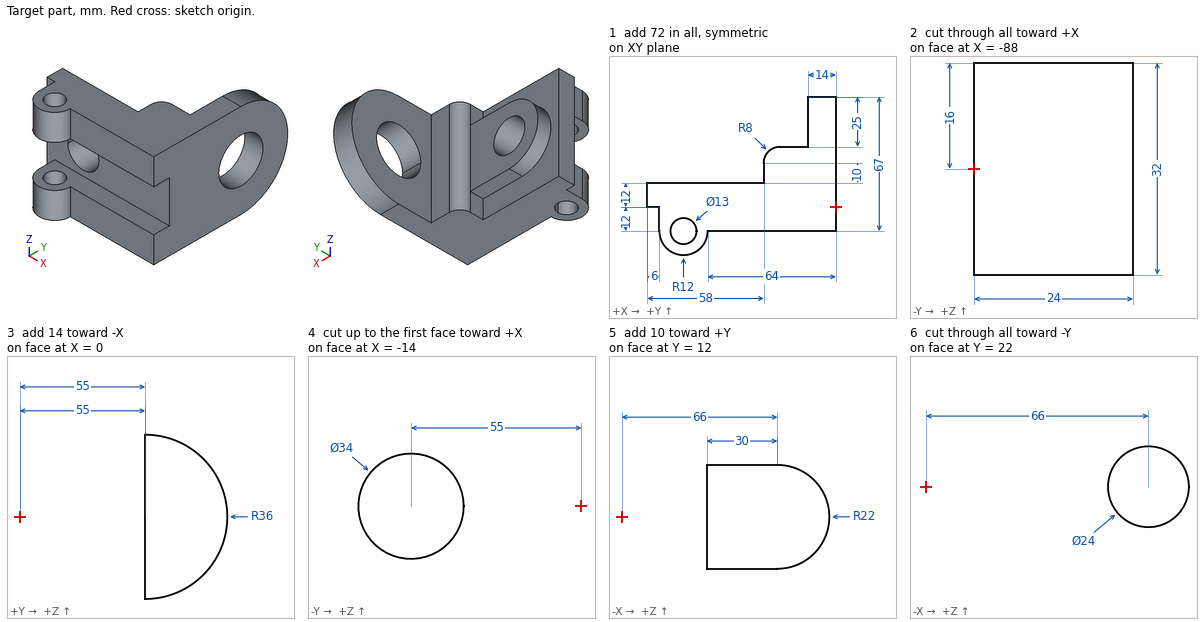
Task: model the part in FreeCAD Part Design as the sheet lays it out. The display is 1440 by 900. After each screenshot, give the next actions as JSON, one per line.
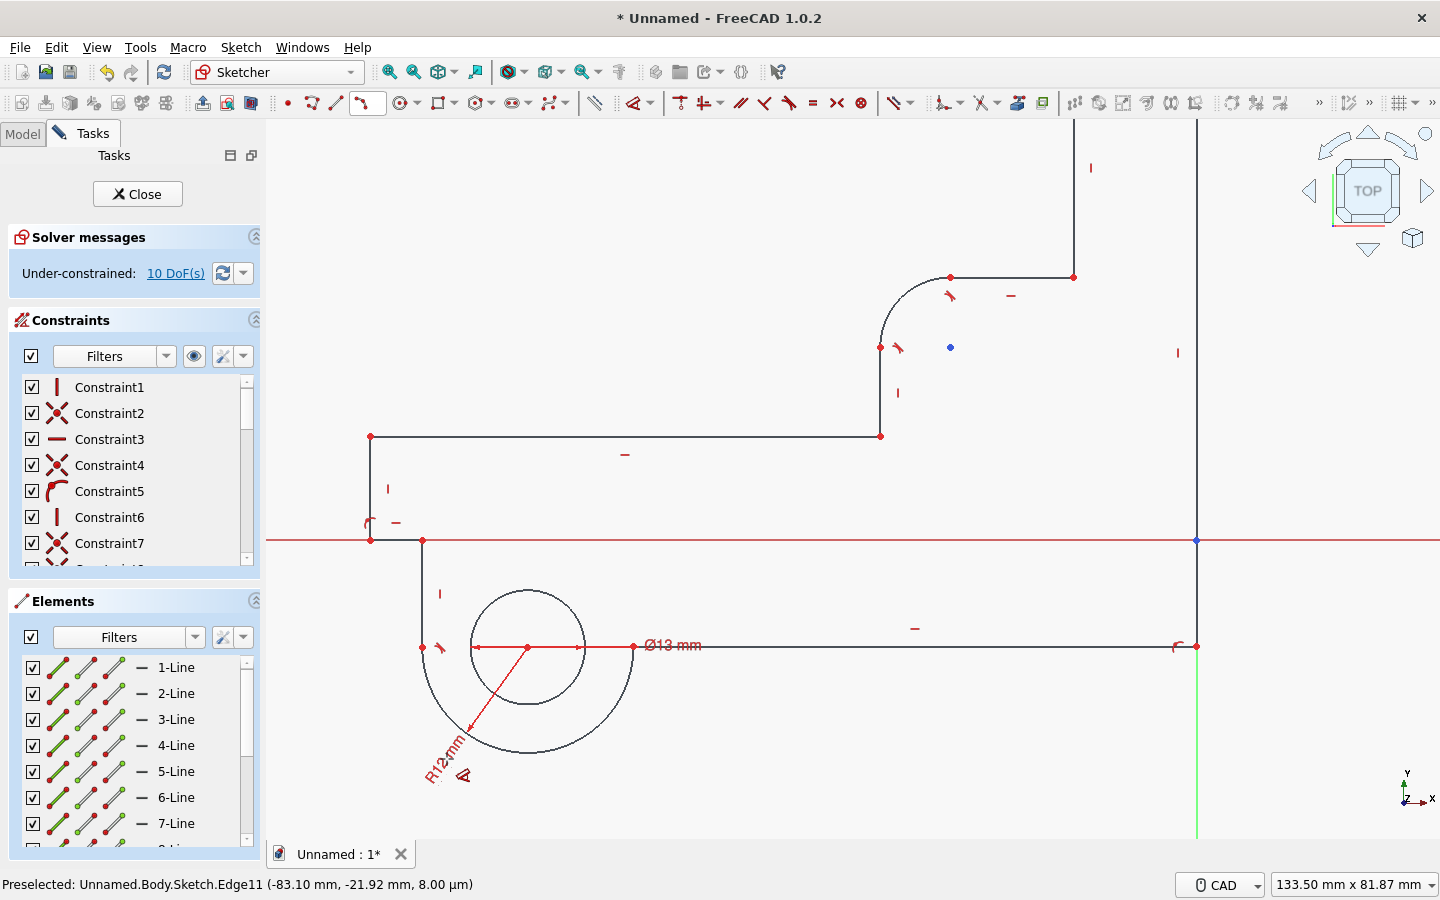
{"action": "left_click", "coordinate": [918, 285]}
{"action": "left_click", "coordinate": [903, 257]}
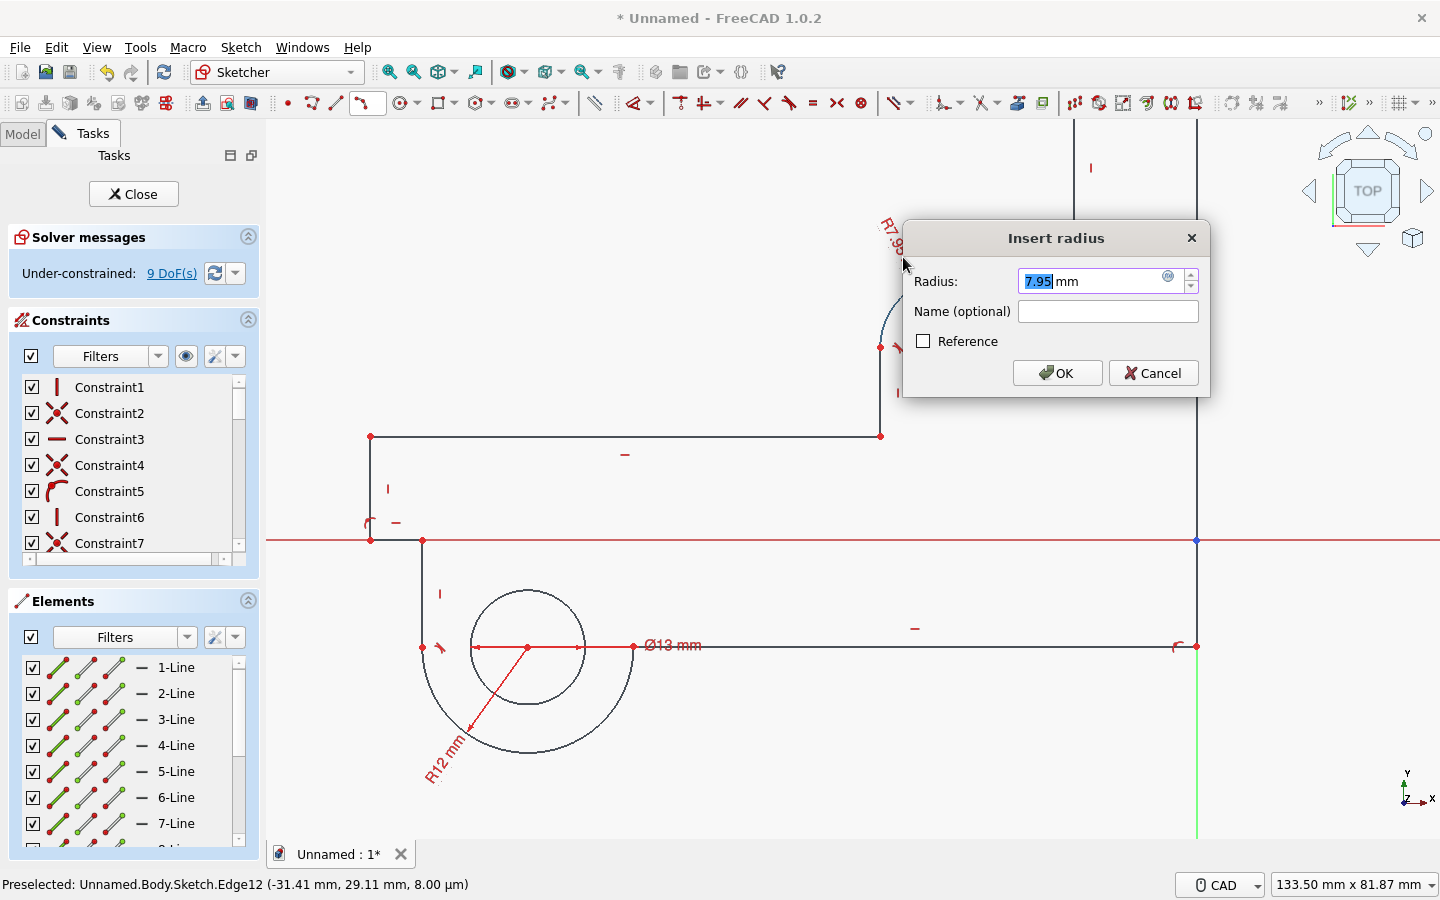
{"action": "type", "text": "8"}
{"action": "key", "text": "Return"}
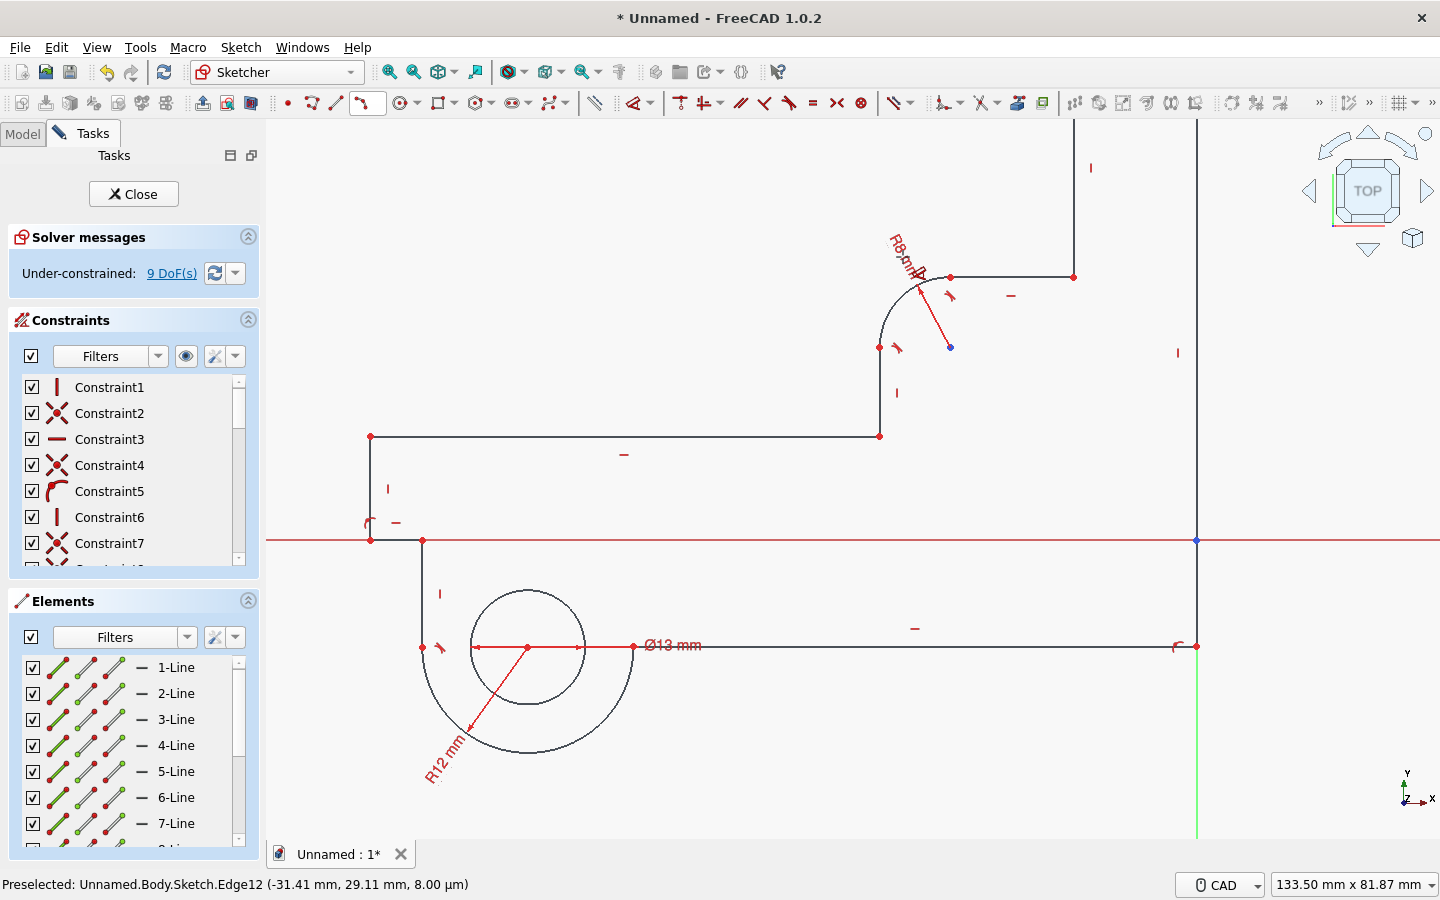
{"action": "left_click", "coordinate": [386, 540]}
{"action": "left_click", "coordinate": [396, 574]}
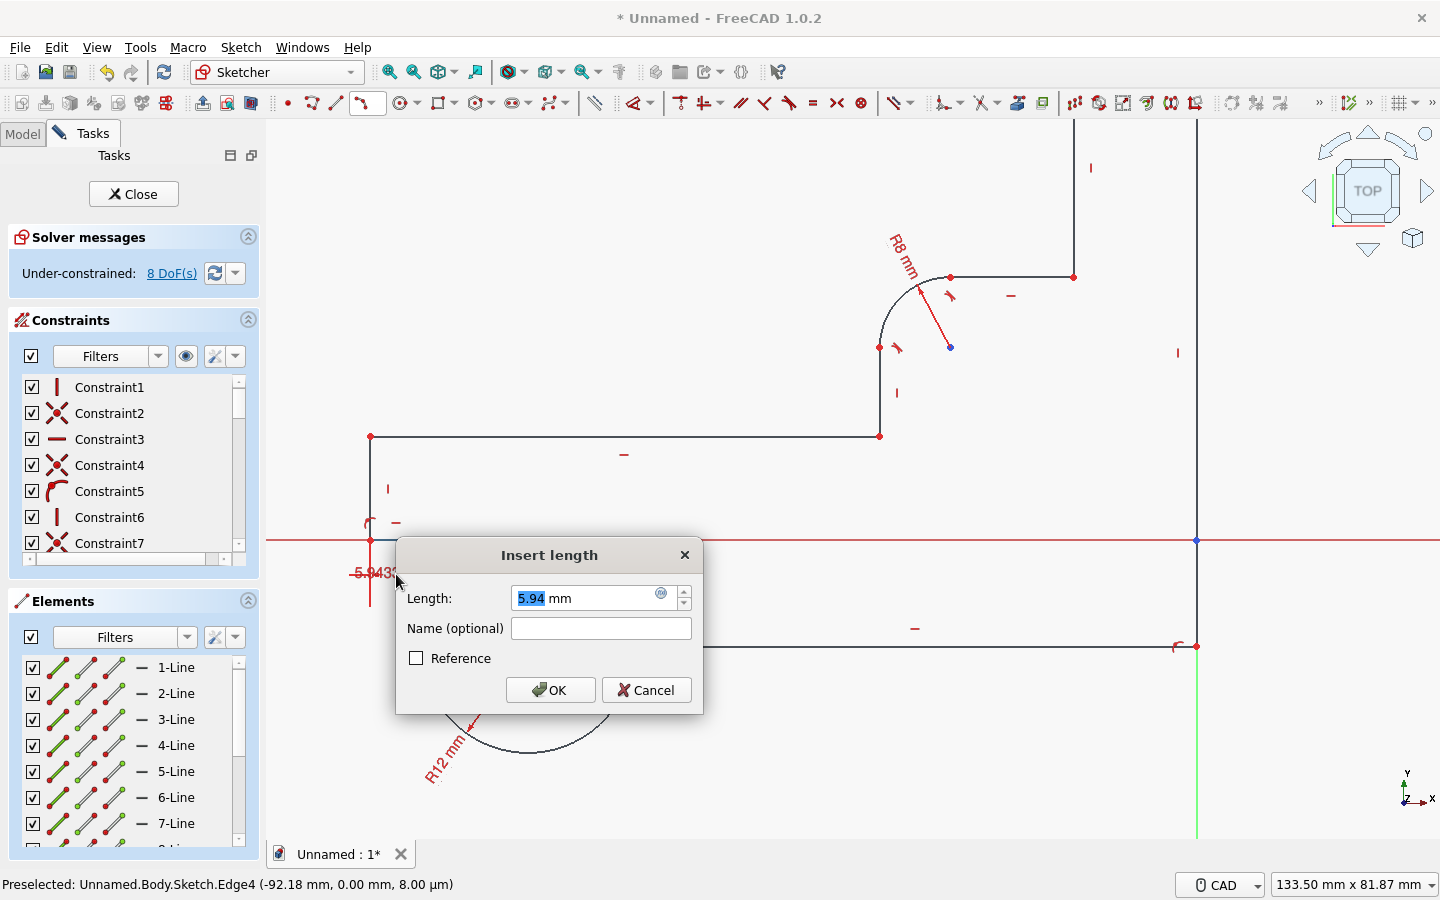
{"action": "type", "text": "6"}
{"action": "key", "text": "Return"}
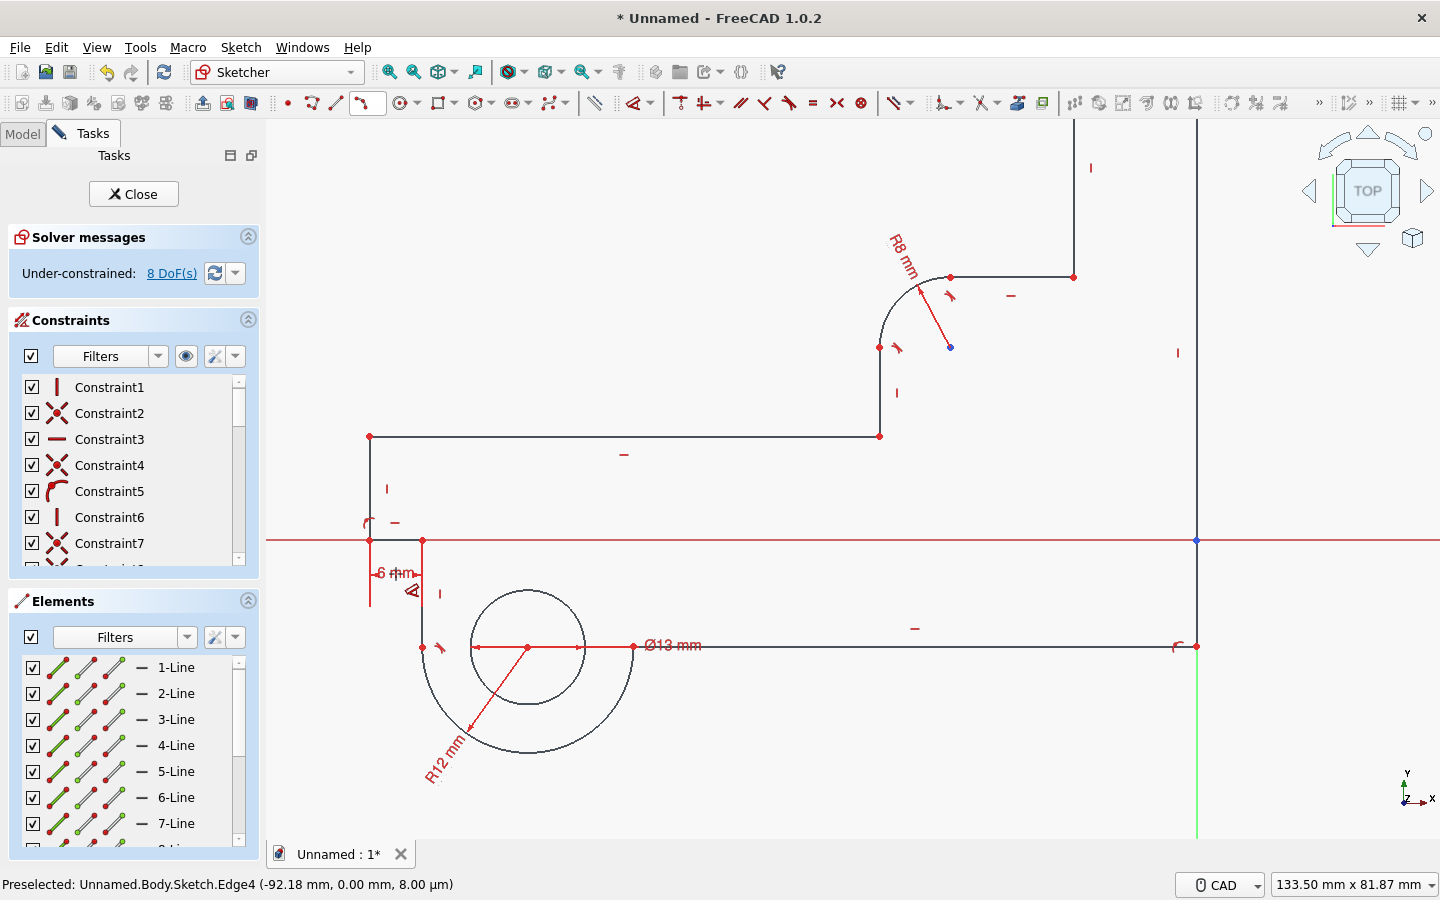
{"action": "left_click", "coordinate": [880, 374]}
{"action": "left_click", "coordinate": [914, 392]}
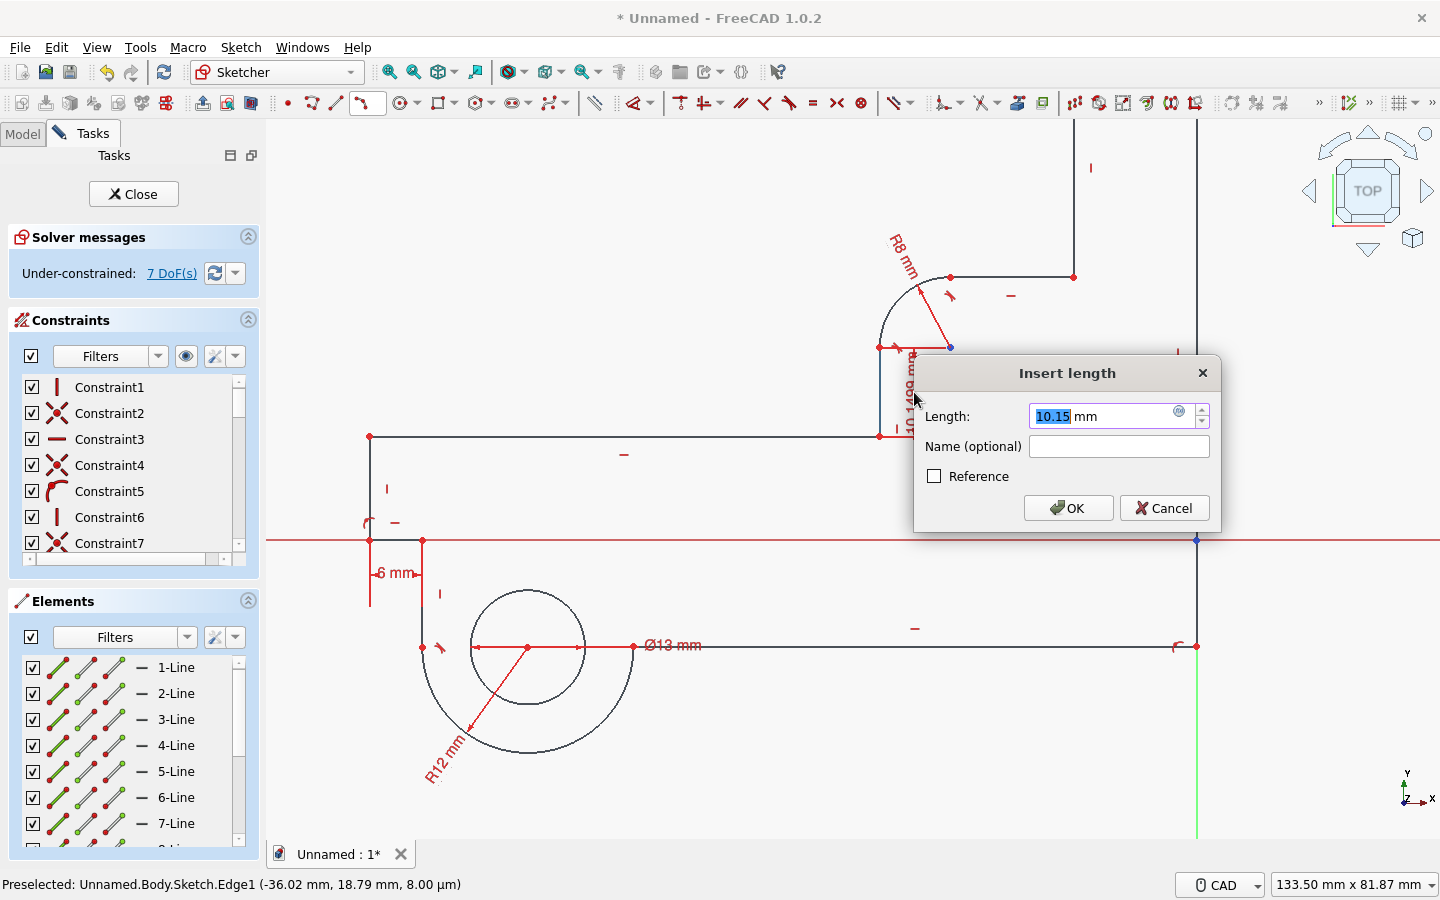
{"action": "type", "text": "10"}
{"action": "key", "text": "Return"}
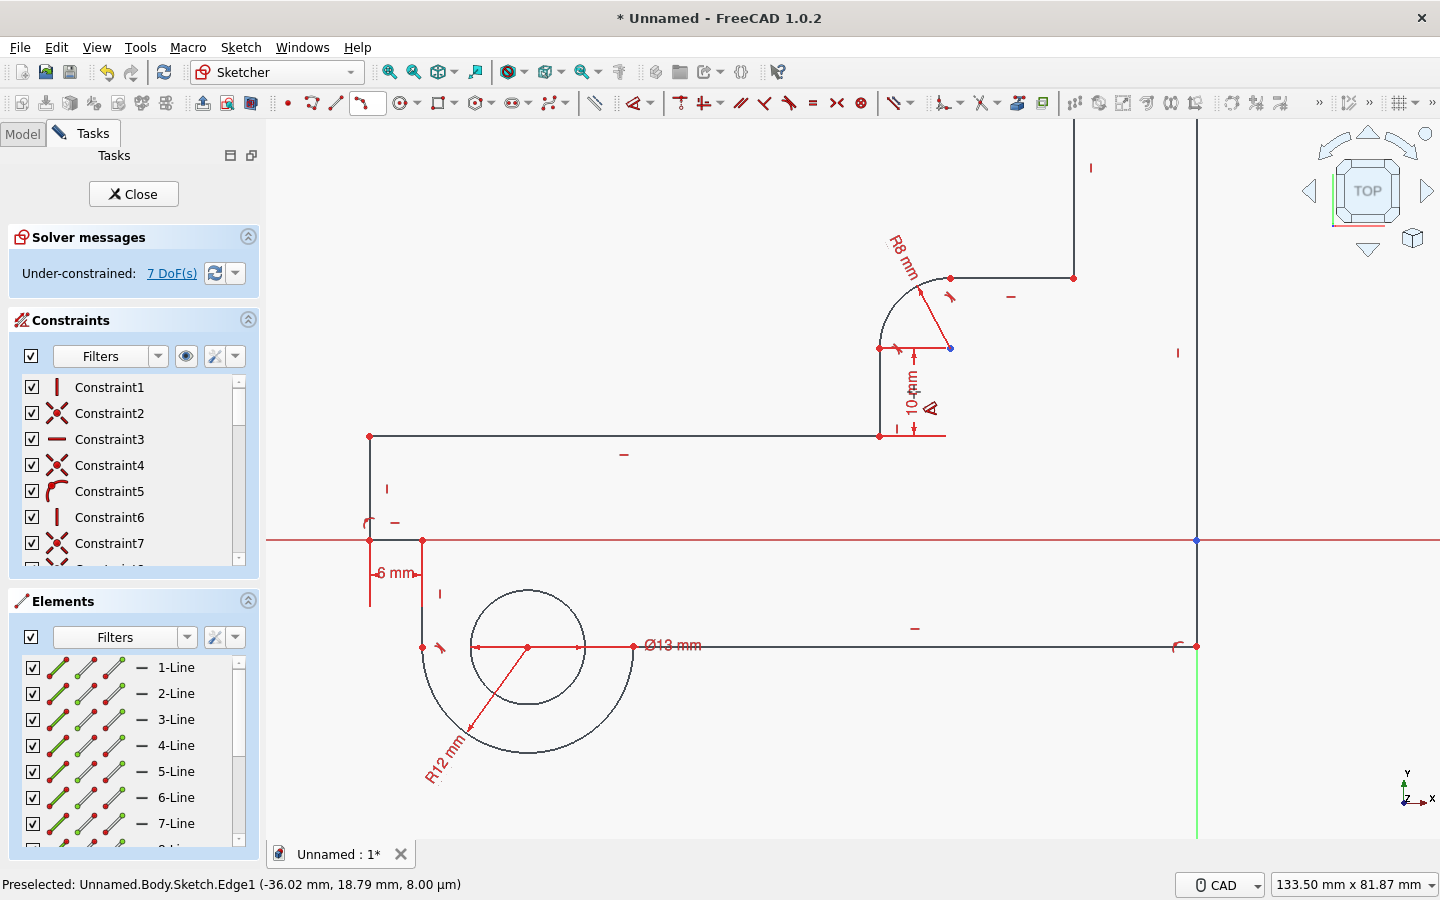
{"action": "left_click", "coordinate": [727, 436]}
{"action": "left_click", "coordinate": [625, 470]}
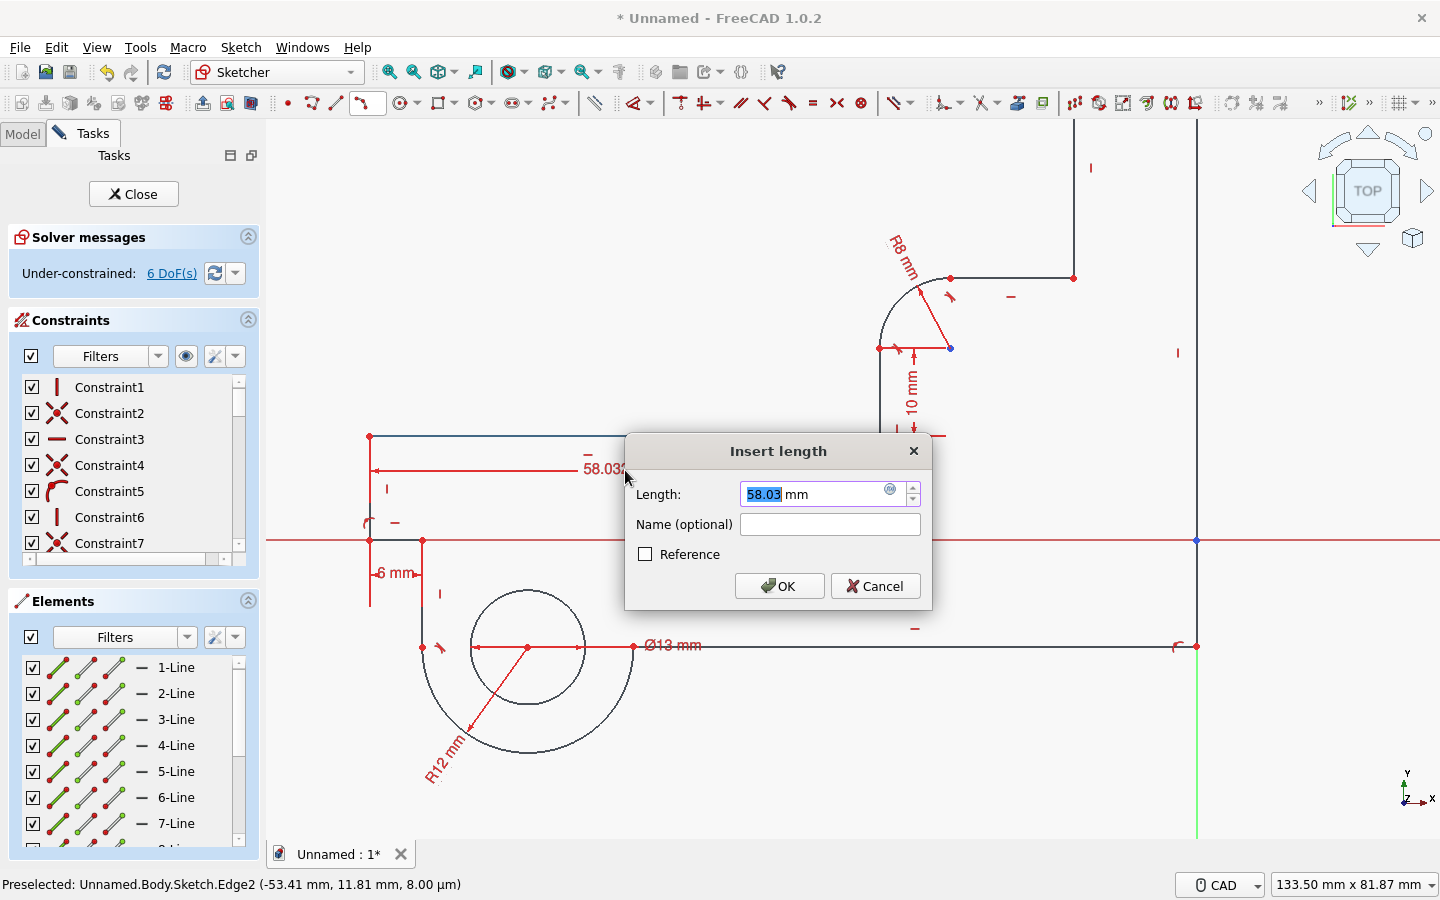
{"action": "type", "text": "58"}
{"action": "key", "text": "Return"}